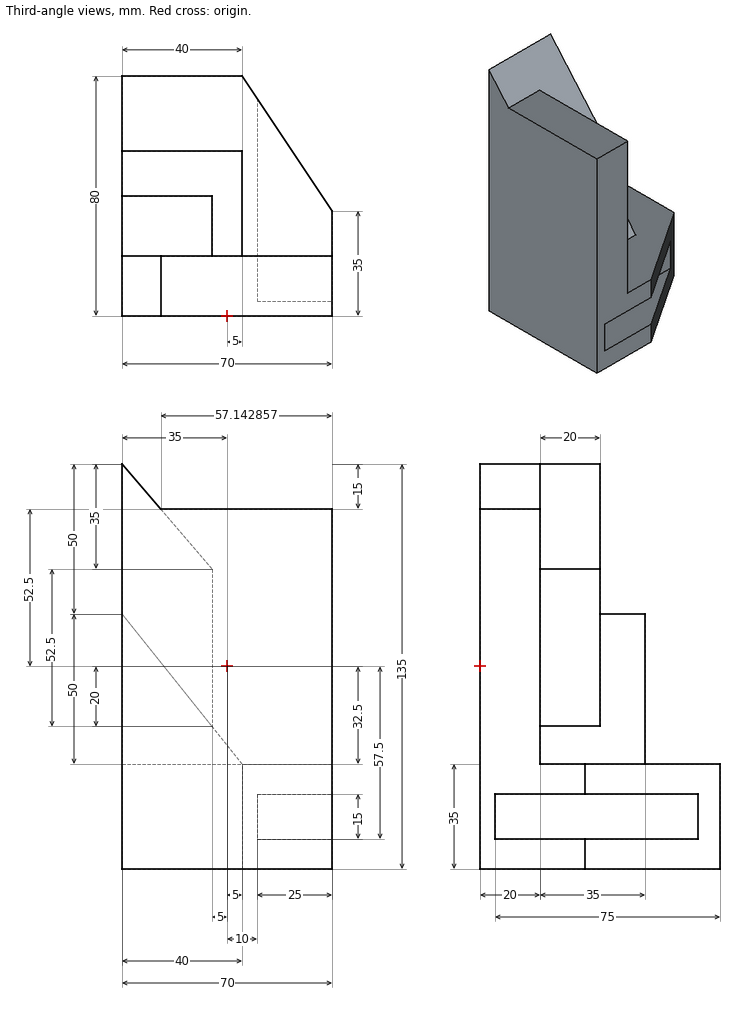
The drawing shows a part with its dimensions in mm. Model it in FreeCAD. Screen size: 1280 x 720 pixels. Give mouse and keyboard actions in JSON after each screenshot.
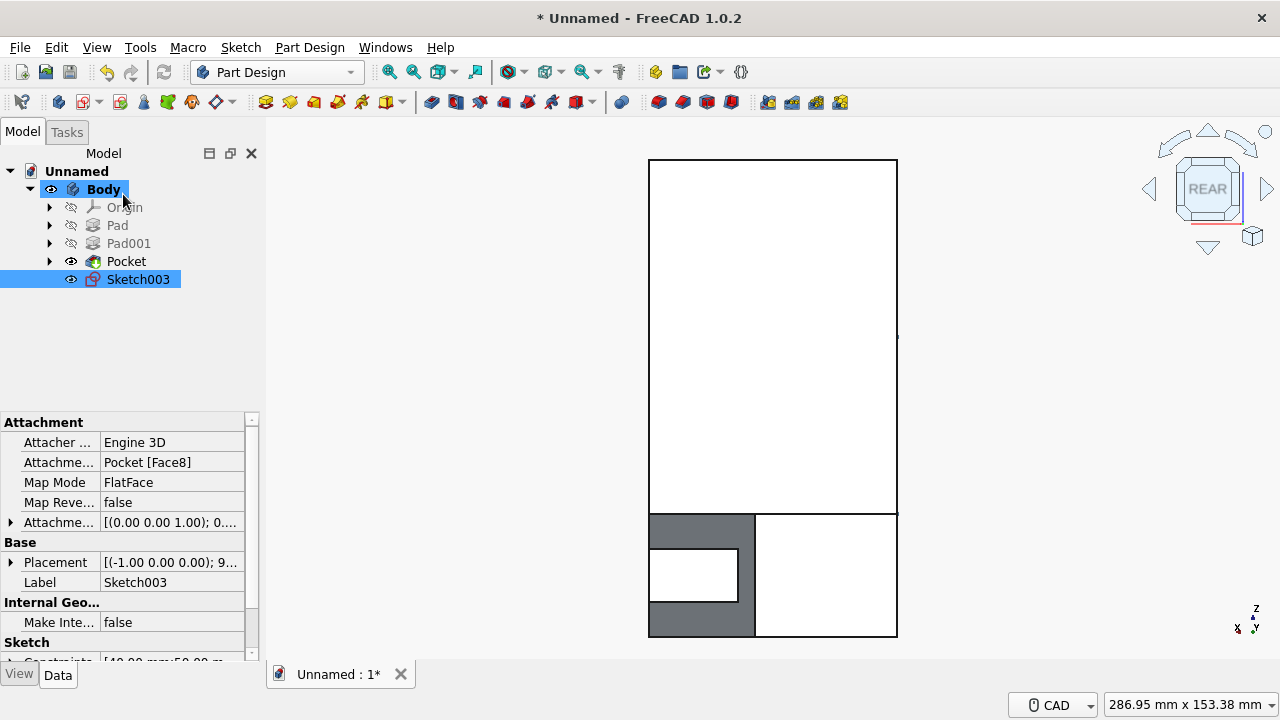
{"action": "left_click", "coordinate": [266, 102]}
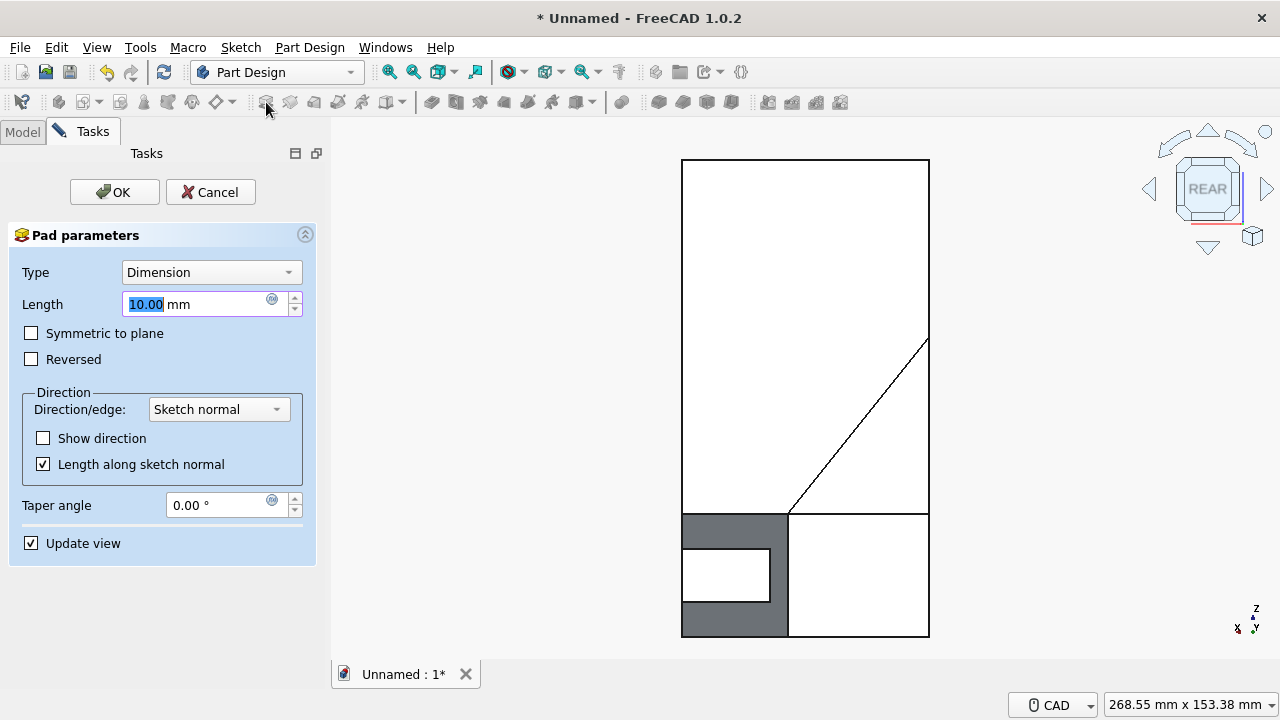
{"action": "type", "text": "35"}
{"action": "key", "text": "Tab"}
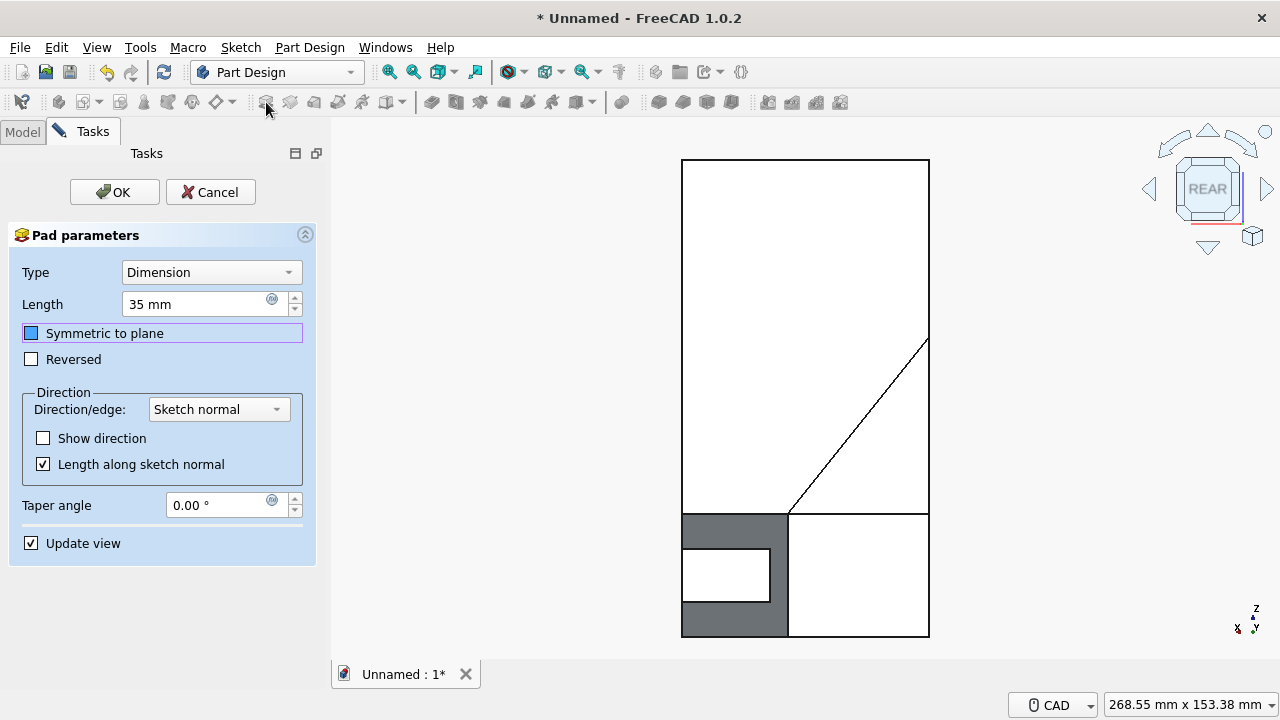
{"action": "left_click", "coordinate": [115, 192]}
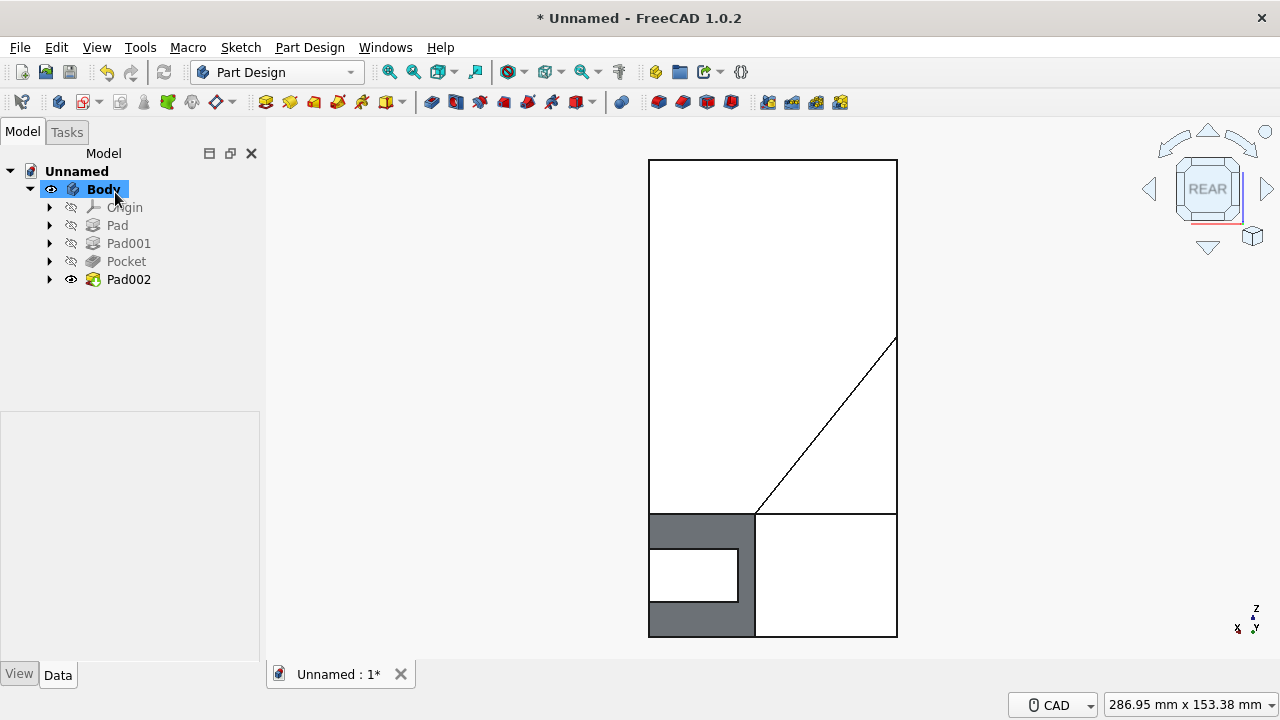
{"action": "left_click", "coordinate": [773, 285]}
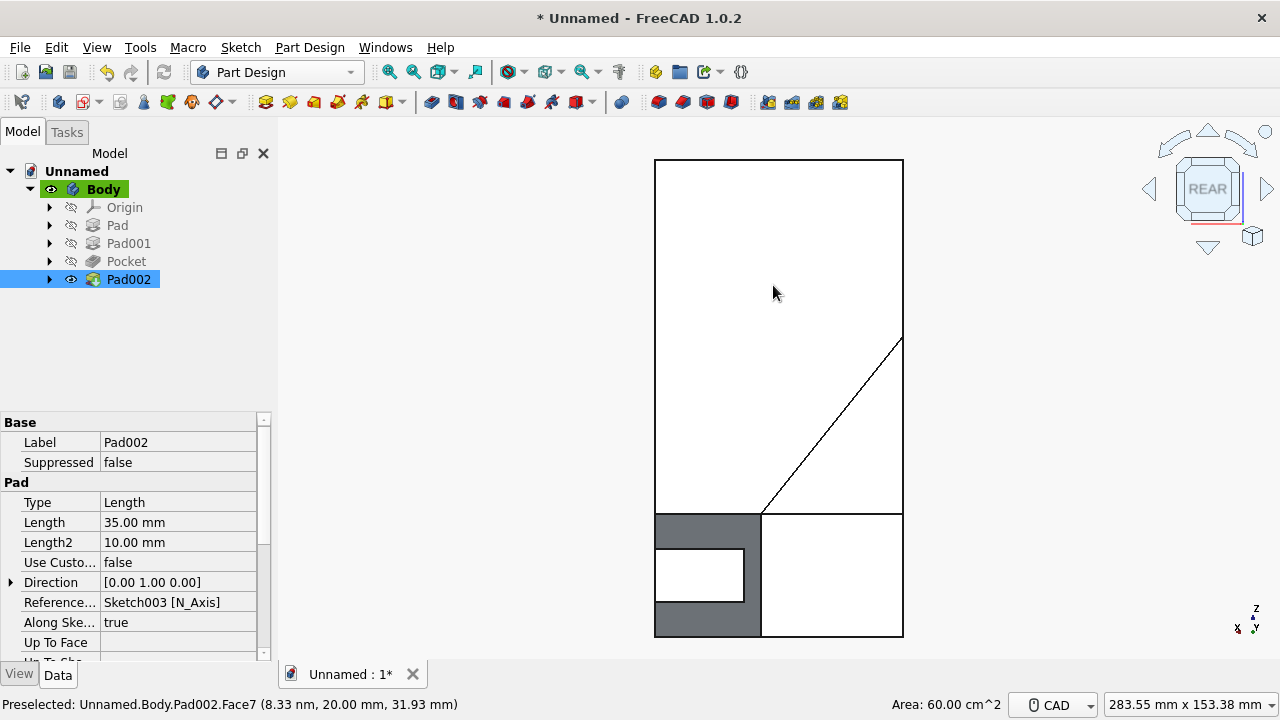
{"action": "left_click", "coordinate": [84, 102]}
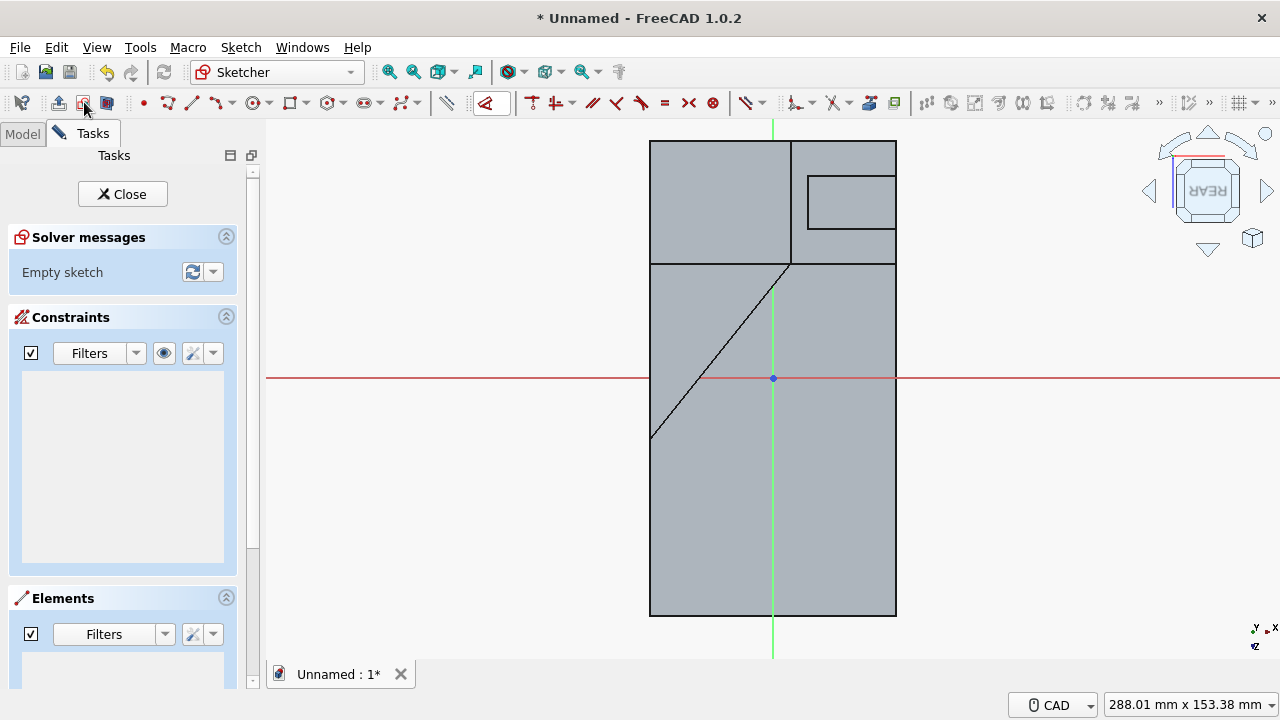
{"action": "left_click", "coordinate": [108, 104]}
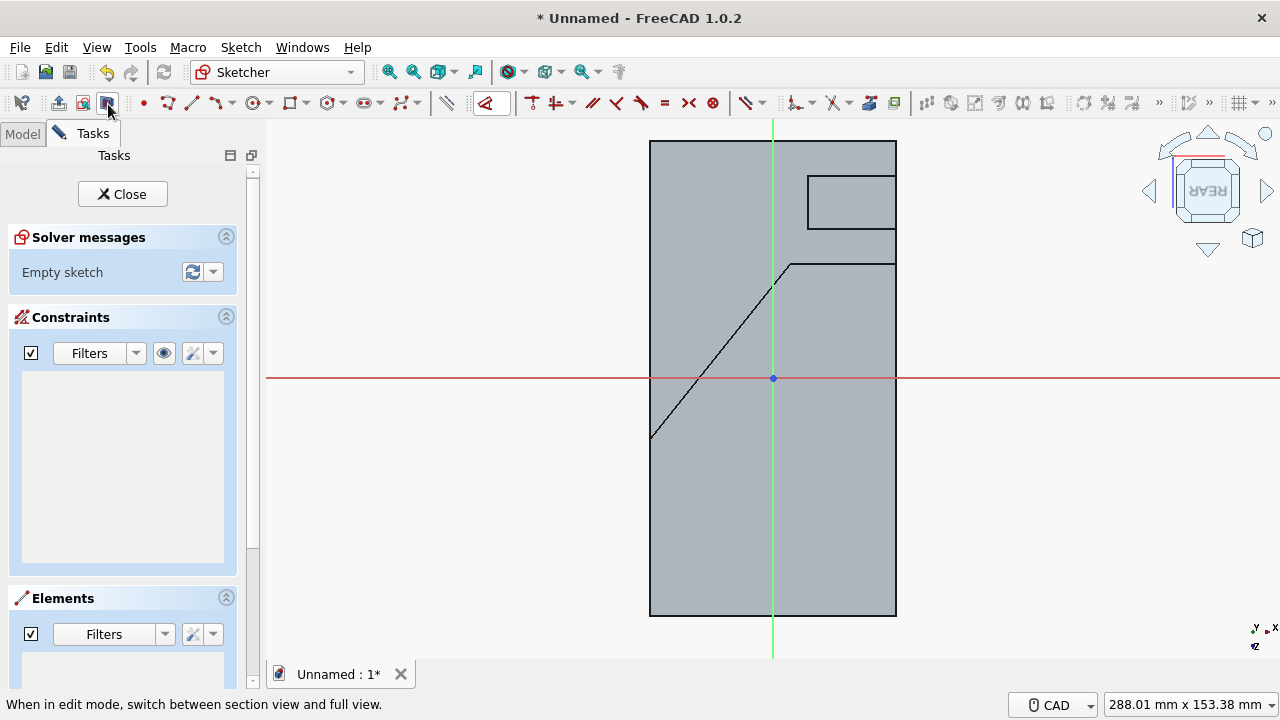
{"action": "scroll", "coordinate": [673, 147], "scroll_direction": "down", "scroll_amount": 1}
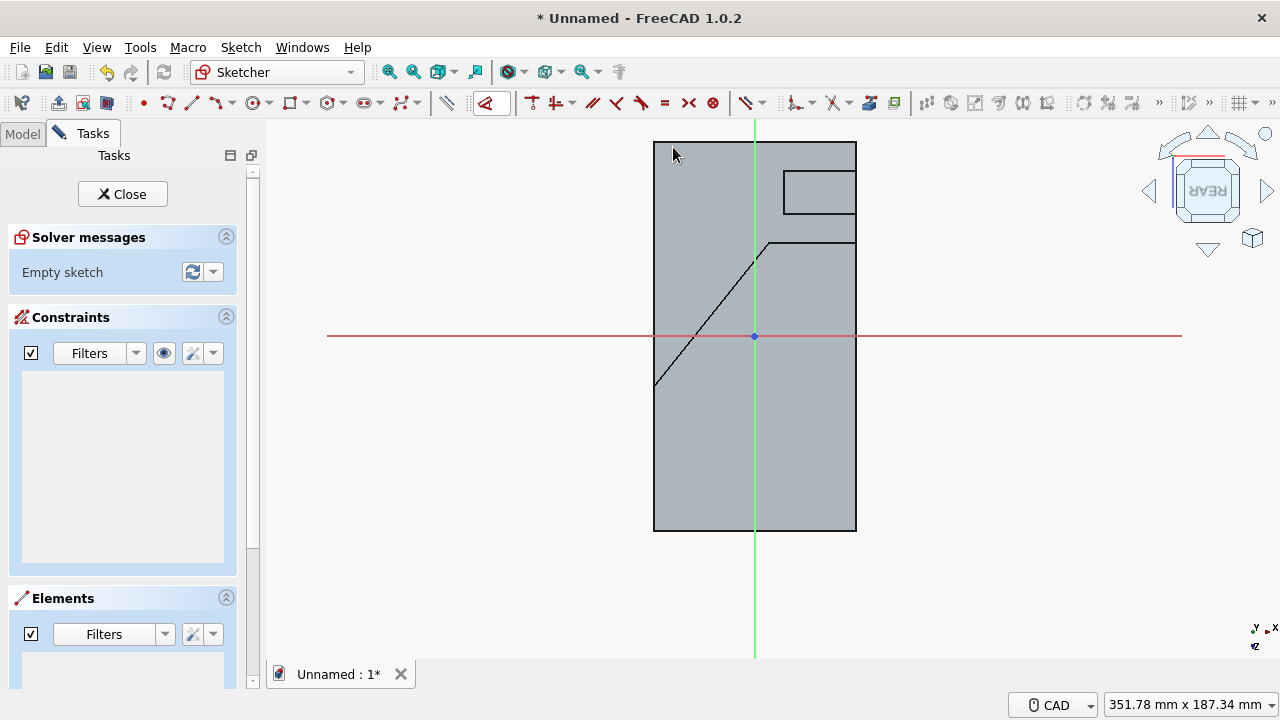
{"action": "scroll", "coordinate": [705, 437], "scroll_direction": "up", "scroll_amount": 2}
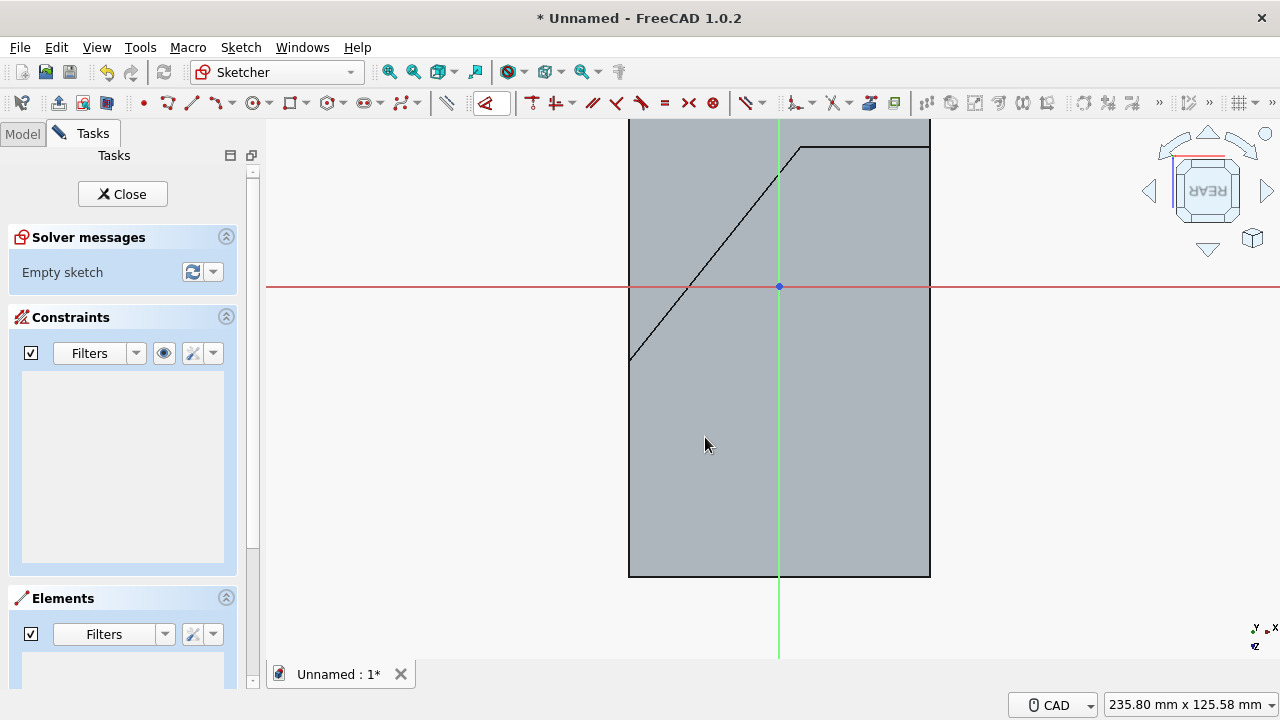
{"action": "left_click", "coordinate": [168, 104]}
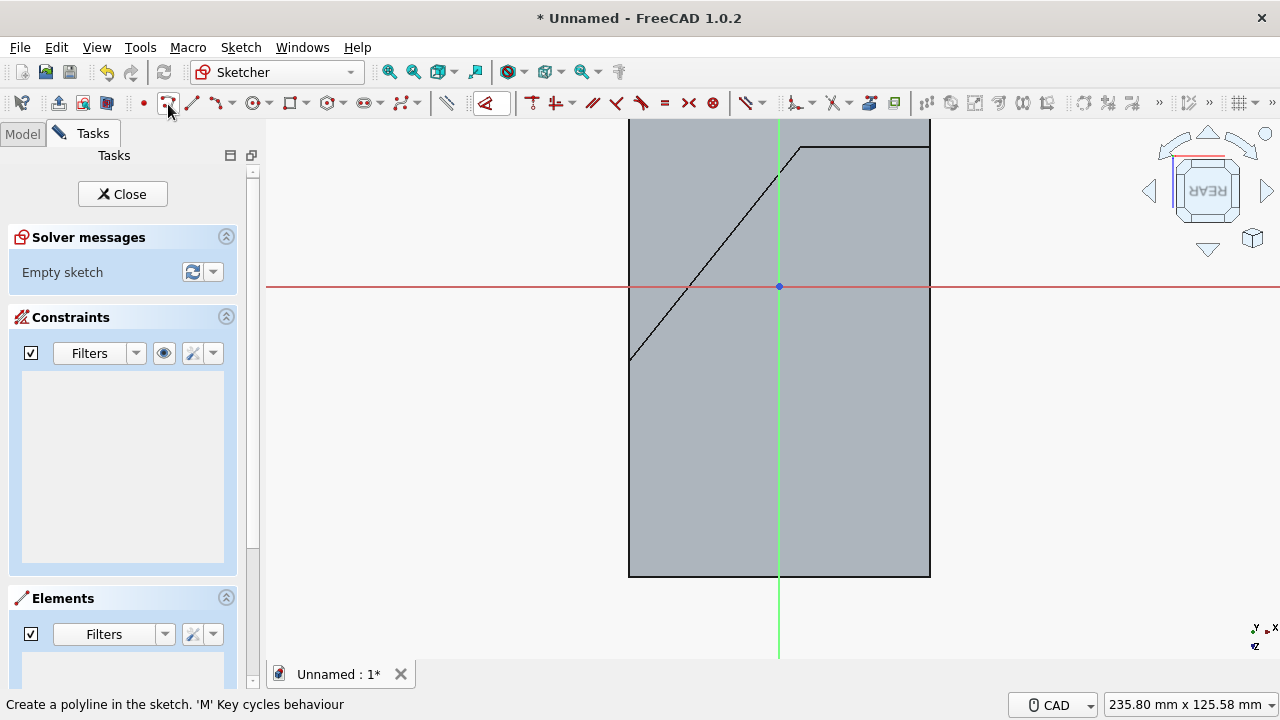
{"action": "left_click", "coordinate": [758, 201]}
{"action": "left_click", "coordinate": [629, 362]}
{"action": "left_click", "coordinate": [629, 577]}
{"action": "left_click", "coordinate": [758, 426]}
{"action": "left_click", "coordinate": [758, 202]}
{"action": "key", "text": "Escape"}
{"action": "key", "text": "Escape"}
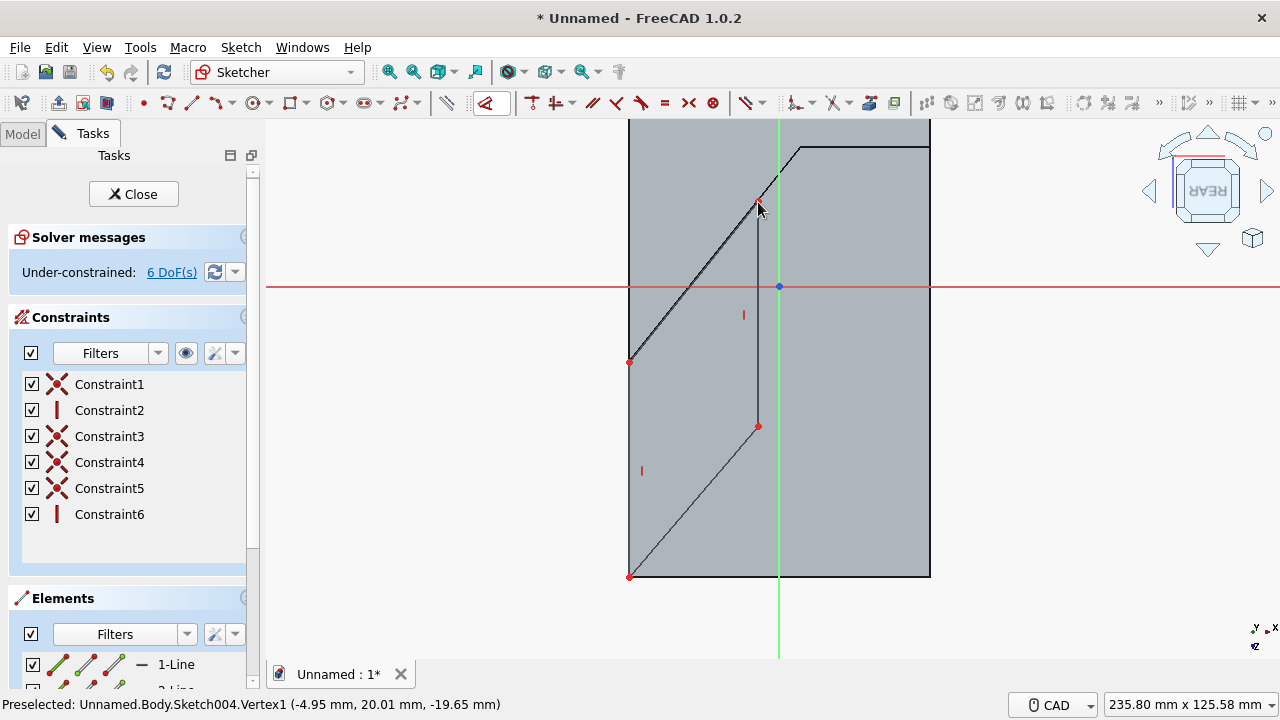
{"action": "left_click", "coordinate": [629, 428]}